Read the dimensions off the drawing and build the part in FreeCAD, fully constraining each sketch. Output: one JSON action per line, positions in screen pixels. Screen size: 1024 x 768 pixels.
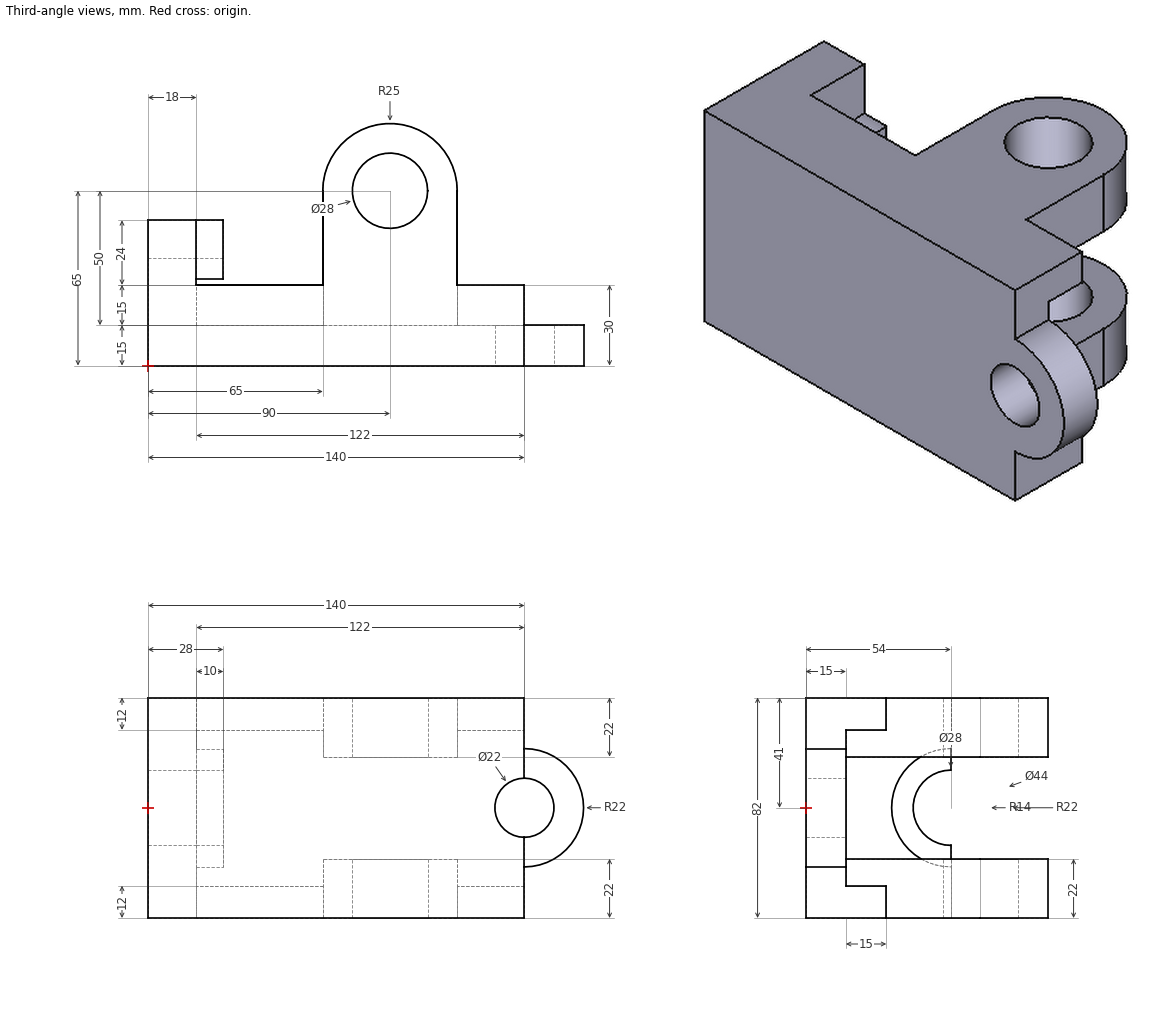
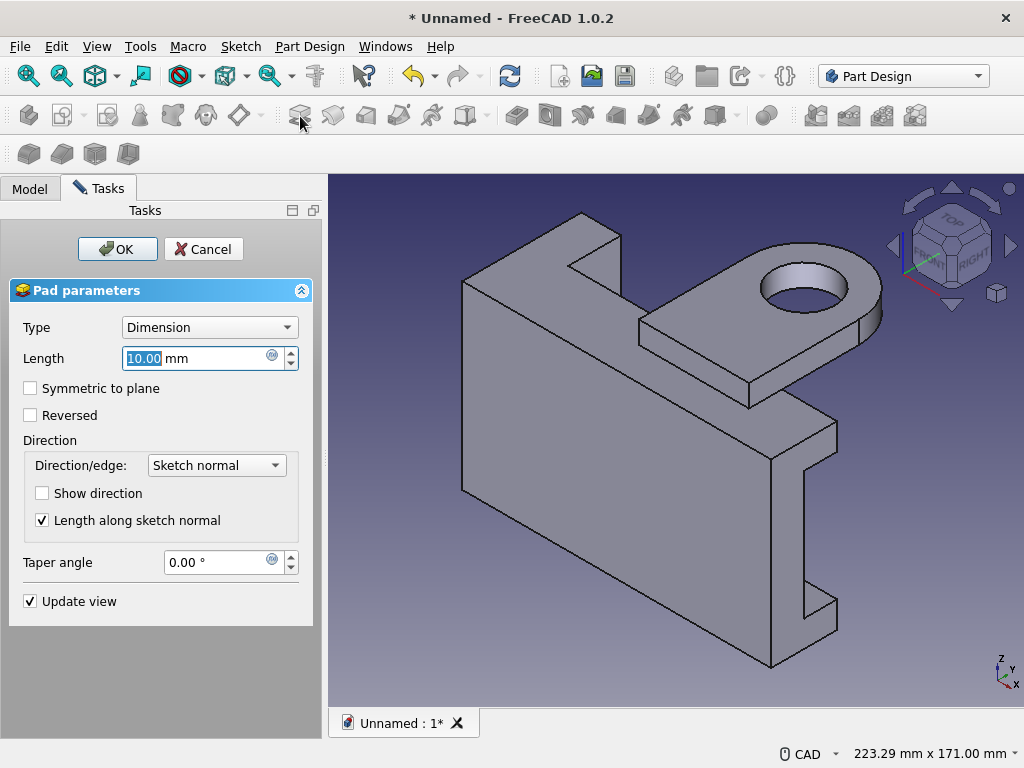
{"action": "type", "text": "22"}
{"action": "key", "text": "Tab"}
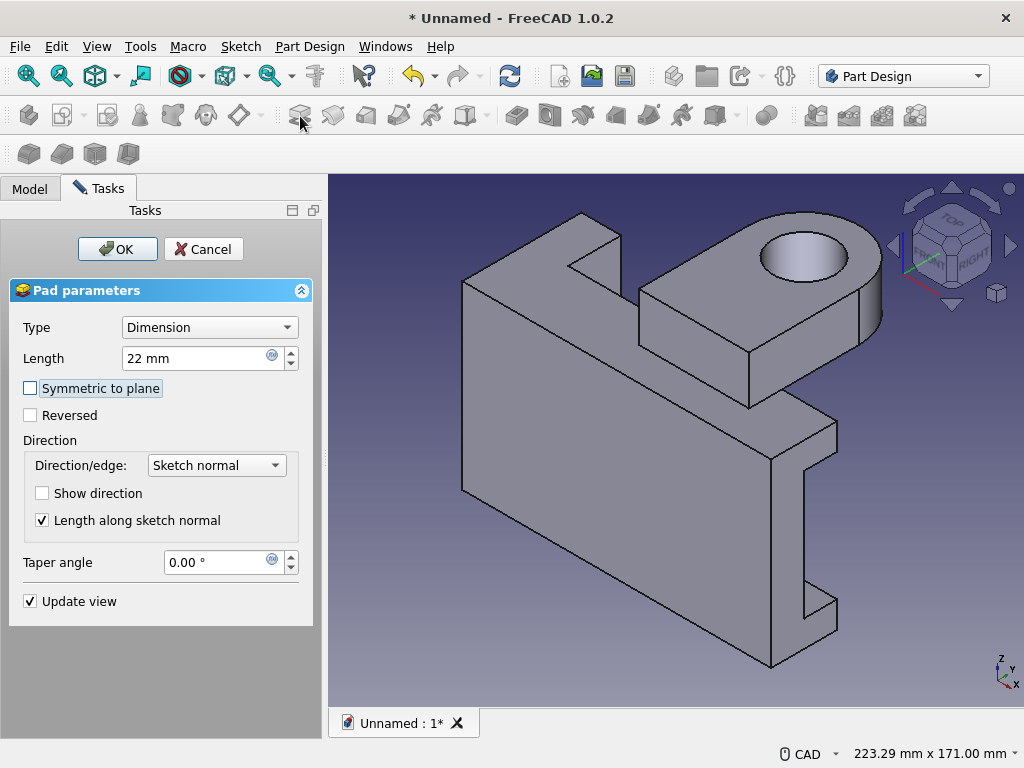
{"action": "left_click", "coordinate": [31, 415]}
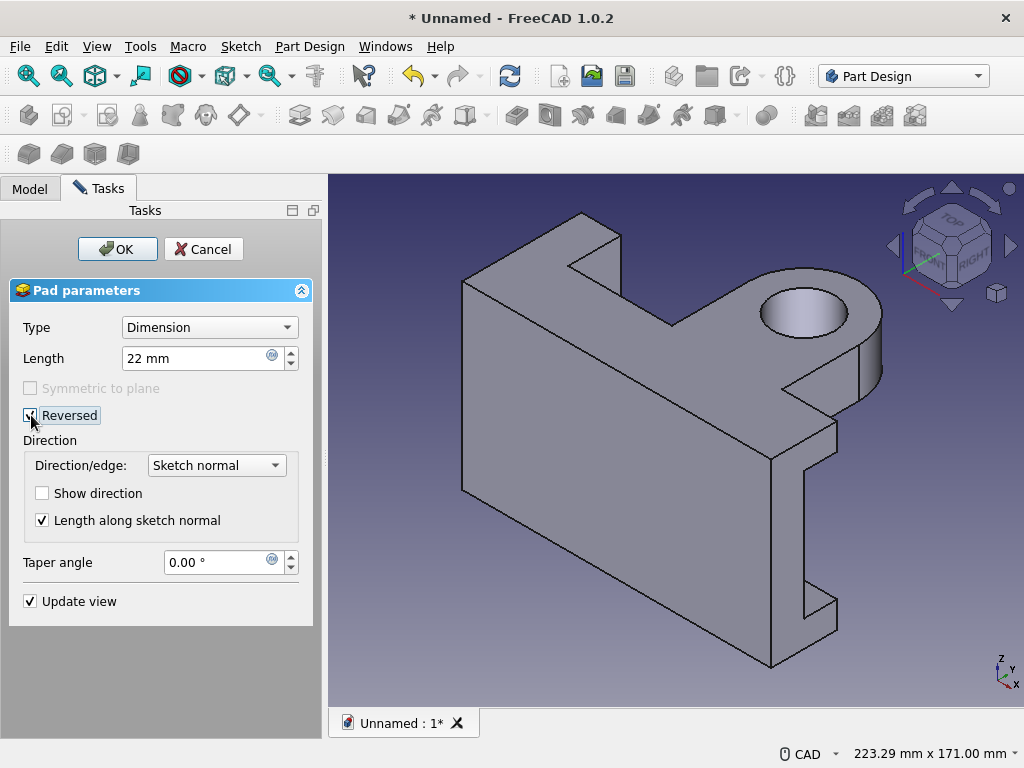
{"action": "left_click", "coordinate": [118, 249]}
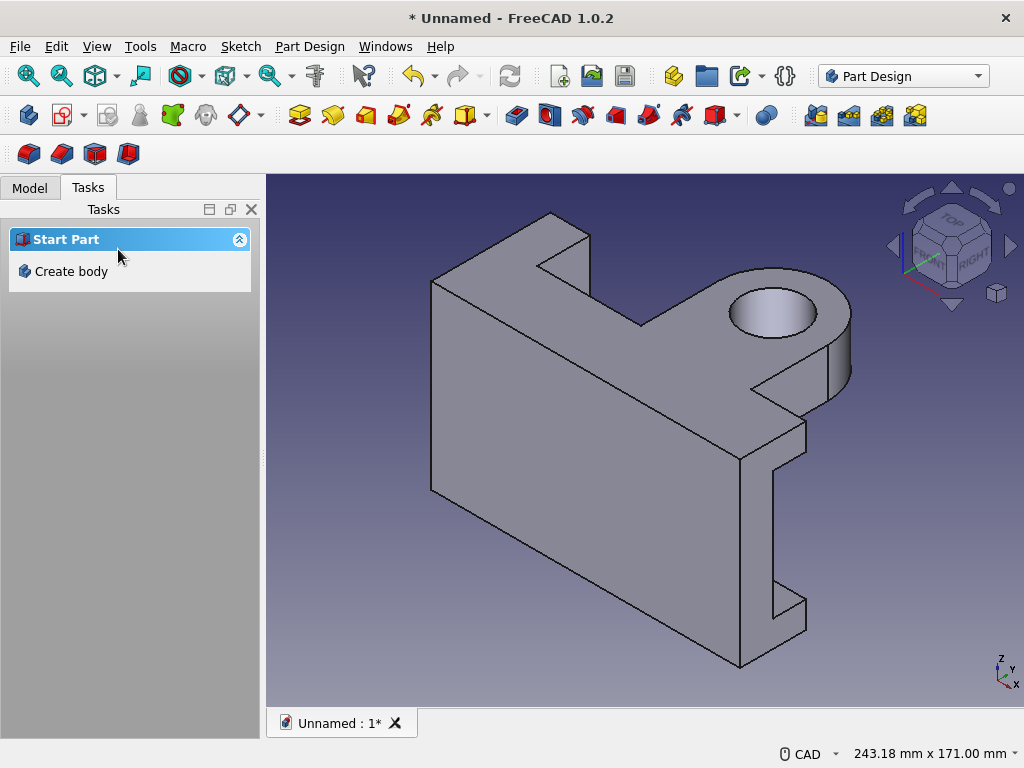
{"action": "key", "text": "v f"}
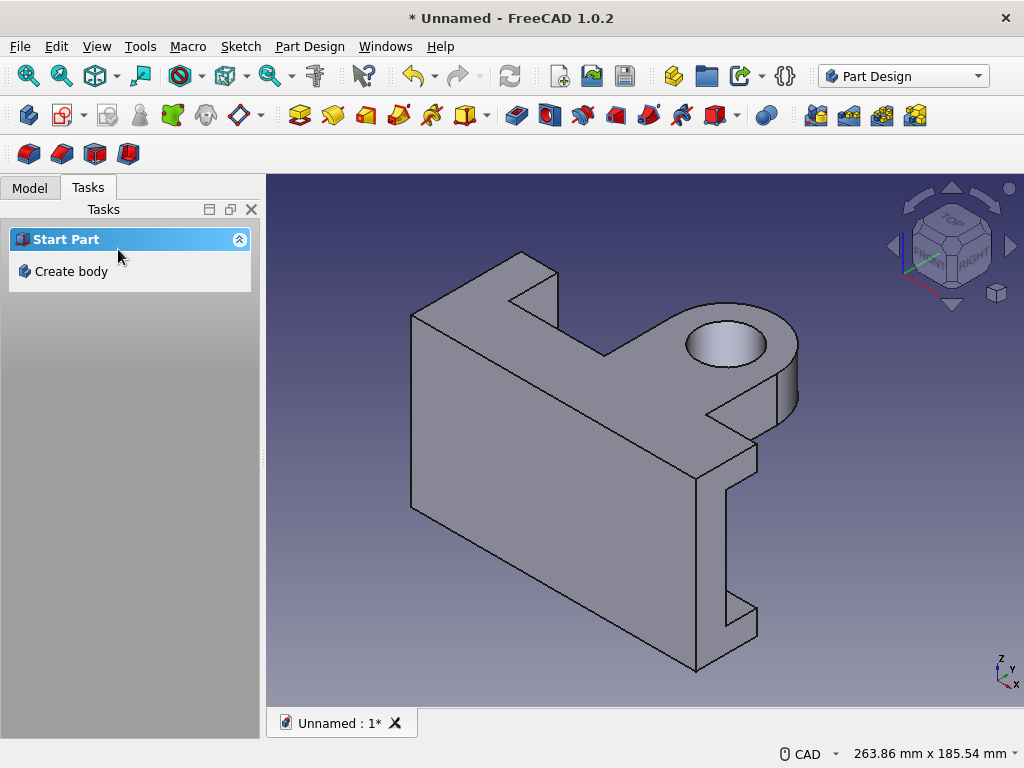
{"action": "left_click", "coordinate": [30, 188]}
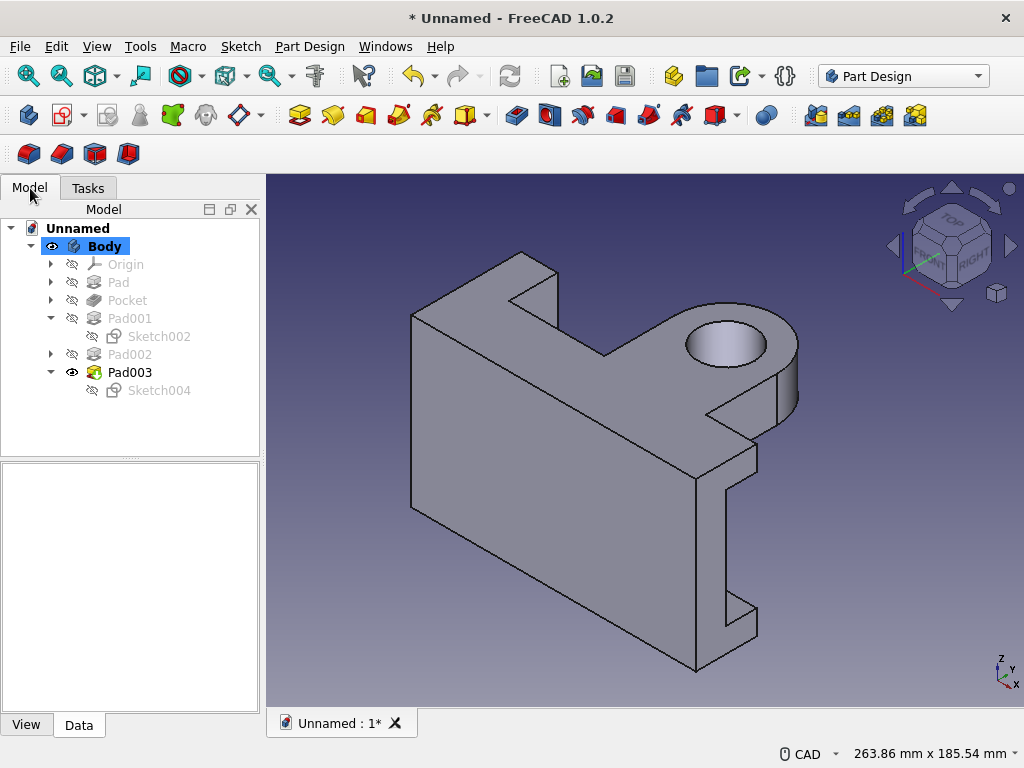
{"action": "left_click", "coordinate": [51, 264]}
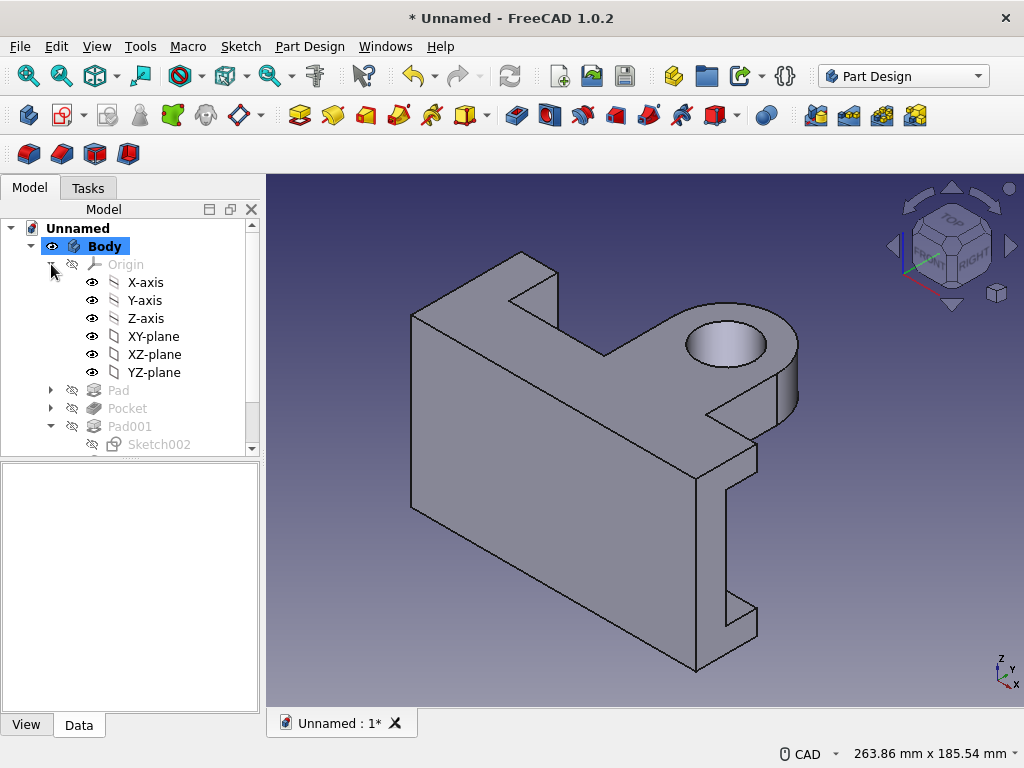
{"action": "left_click", "coordinate": [137, 336]}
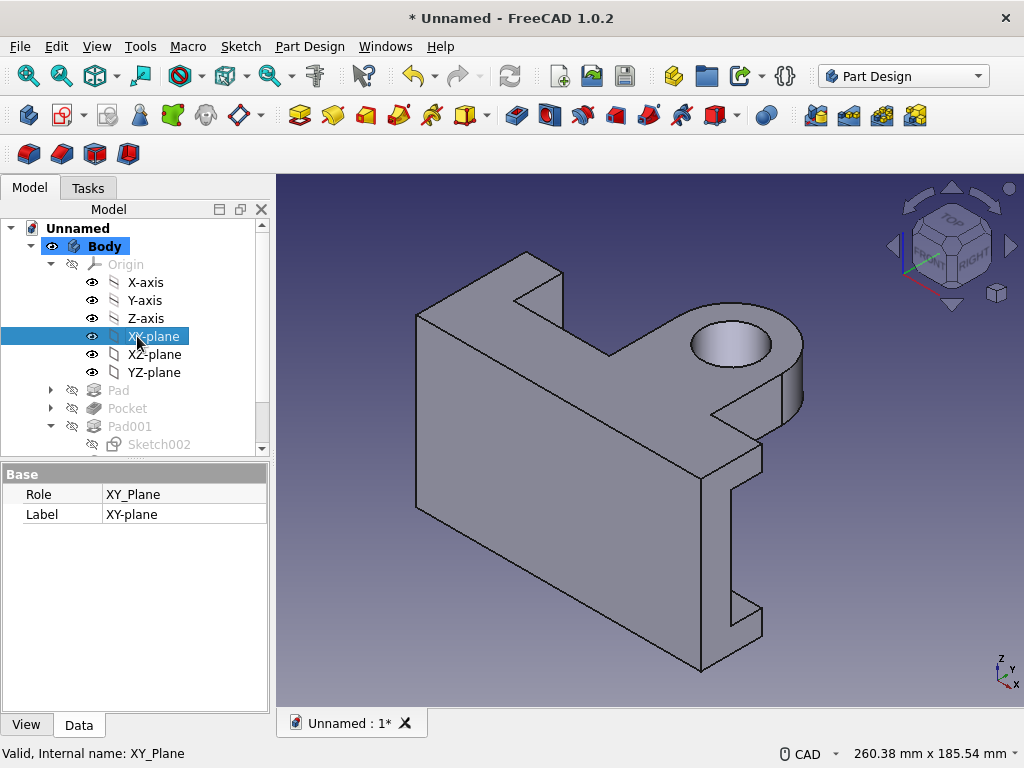
{"action": "left_click", "coordinate": [238, 116]}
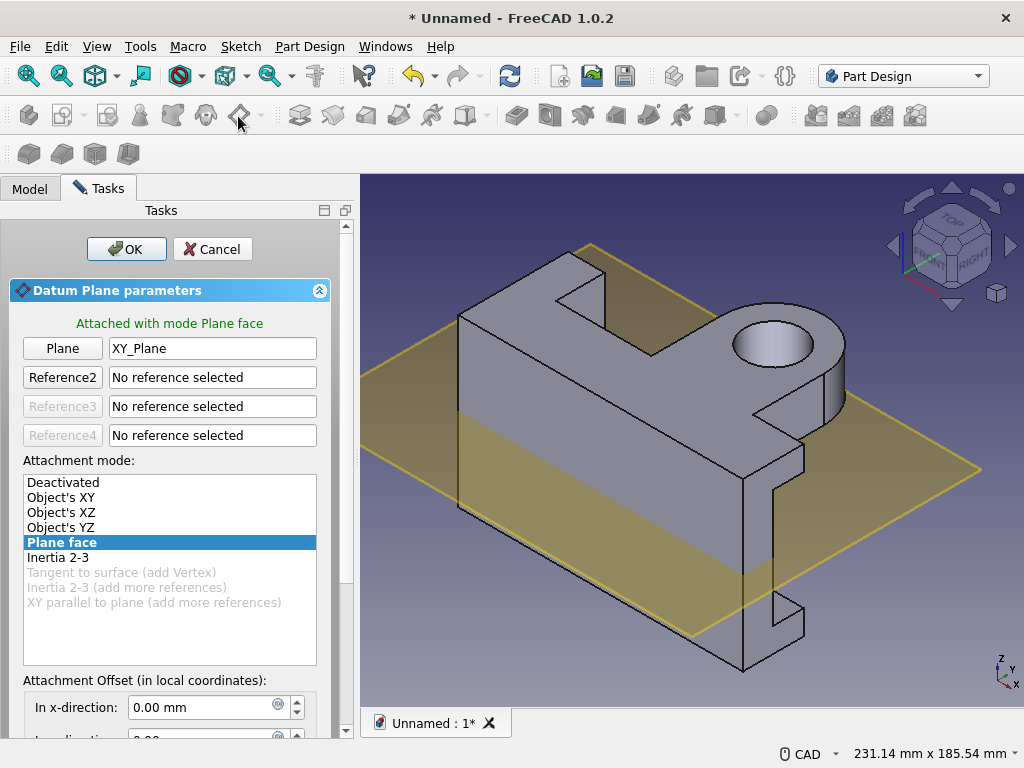
{"action": "scroll", "coordinate": [346, 479], "scroll_direction": "down", "scroll_amount": 2}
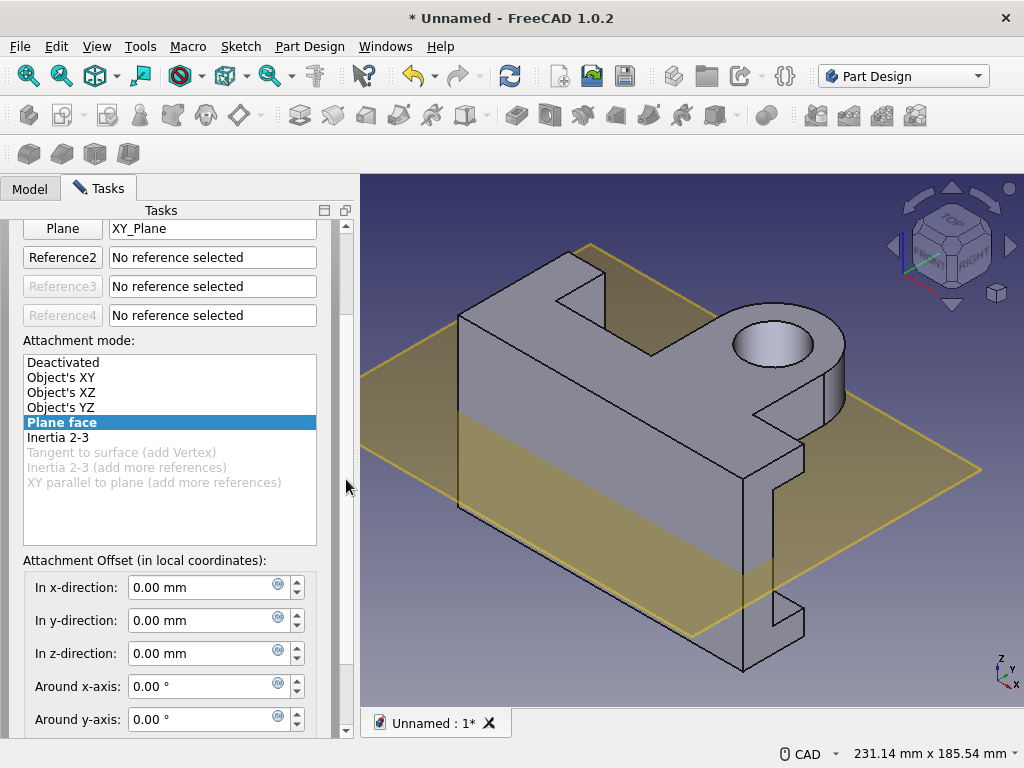
{"action": "triple_click", "coordinate": [210, 654]}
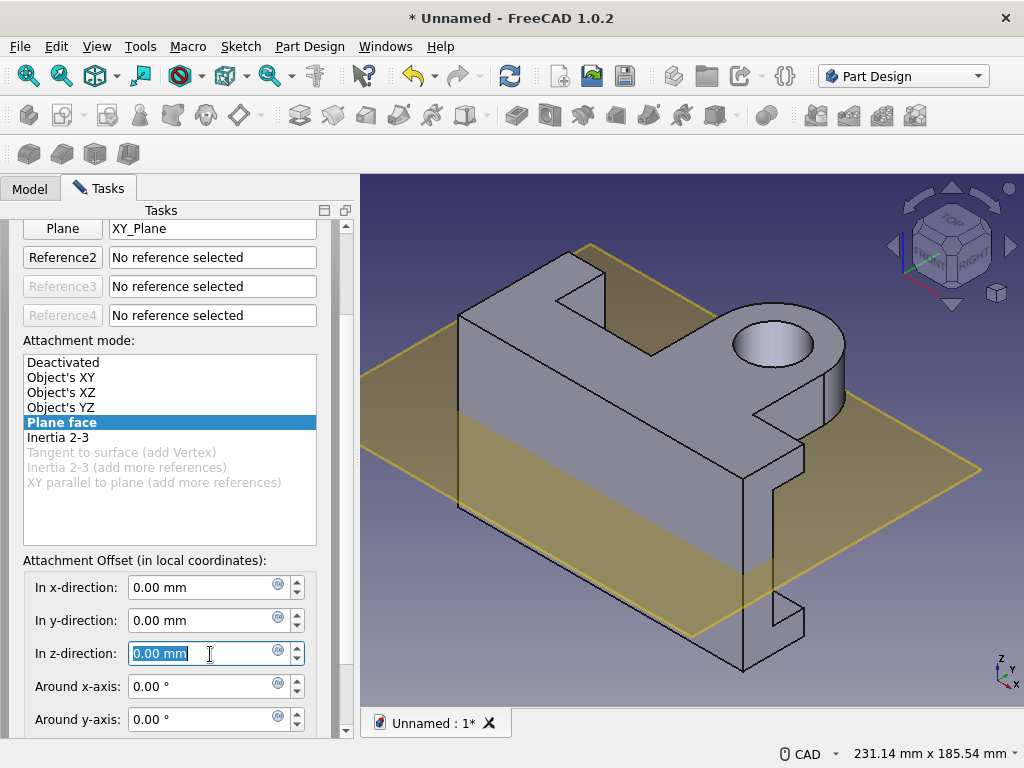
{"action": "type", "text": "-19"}
{"action": "key", "text": "Tab"}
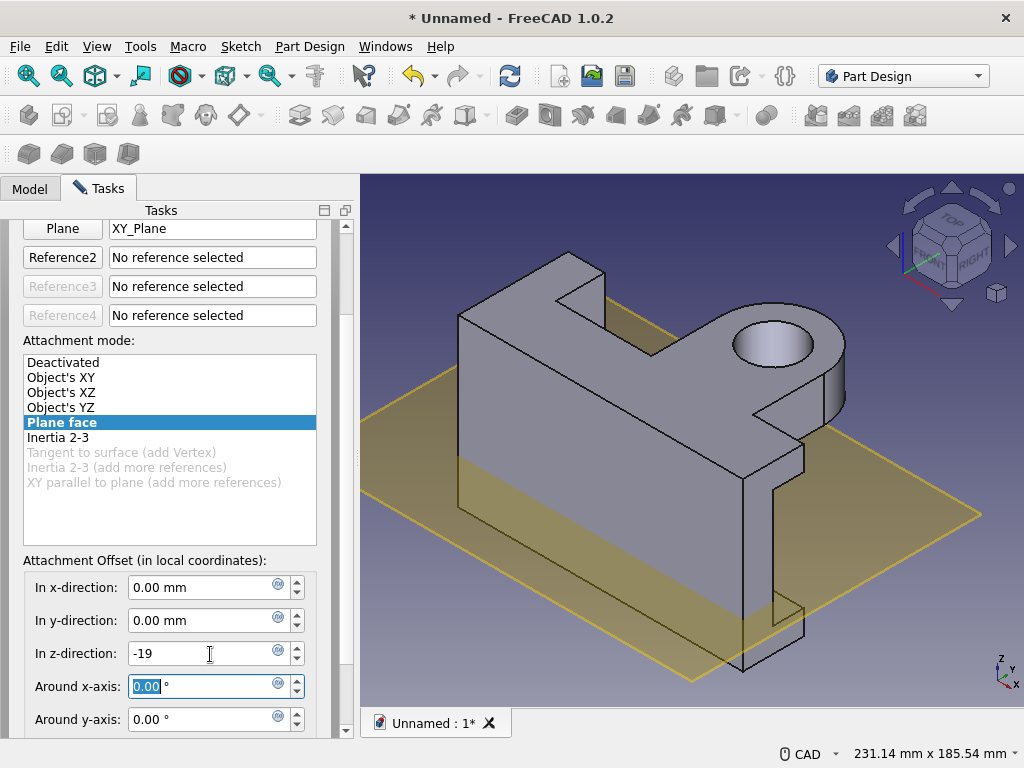
{"action": "scroll", "coordinate": [346, 479], "scroll_direction": "up", "scroll_amount": 3}